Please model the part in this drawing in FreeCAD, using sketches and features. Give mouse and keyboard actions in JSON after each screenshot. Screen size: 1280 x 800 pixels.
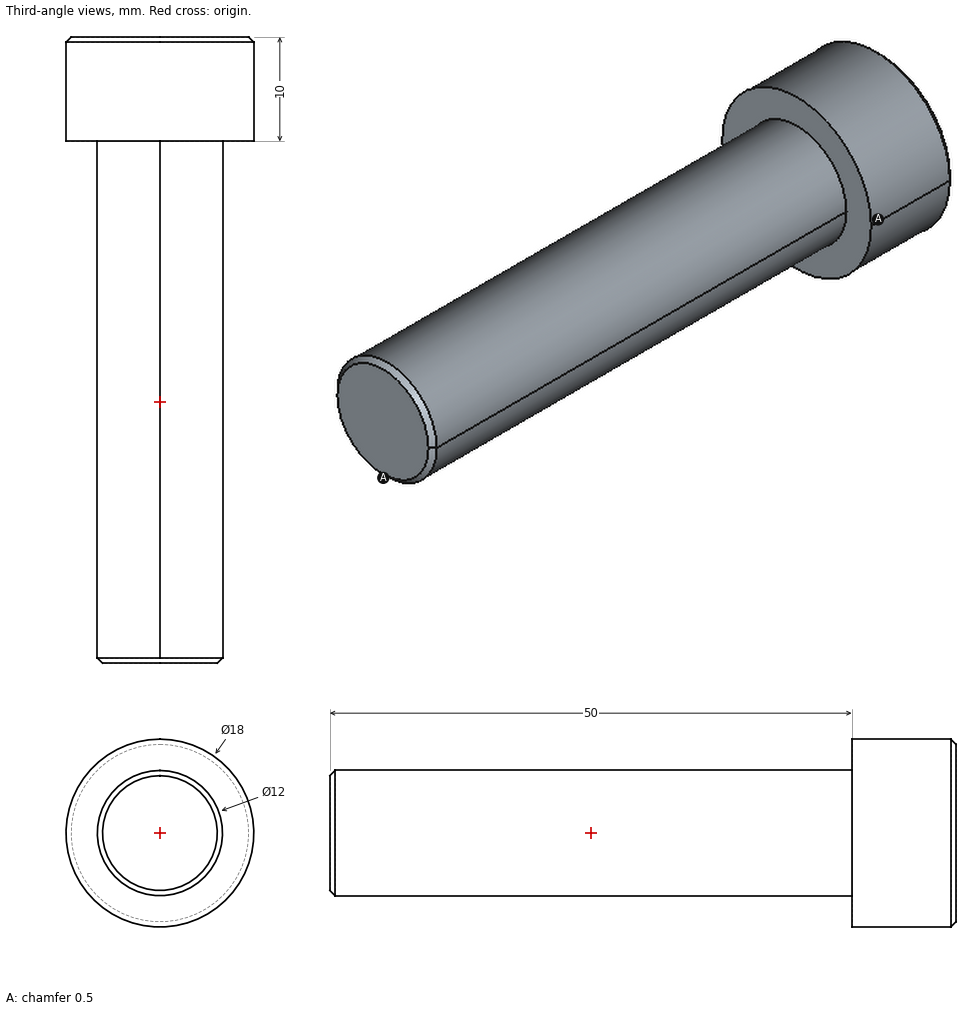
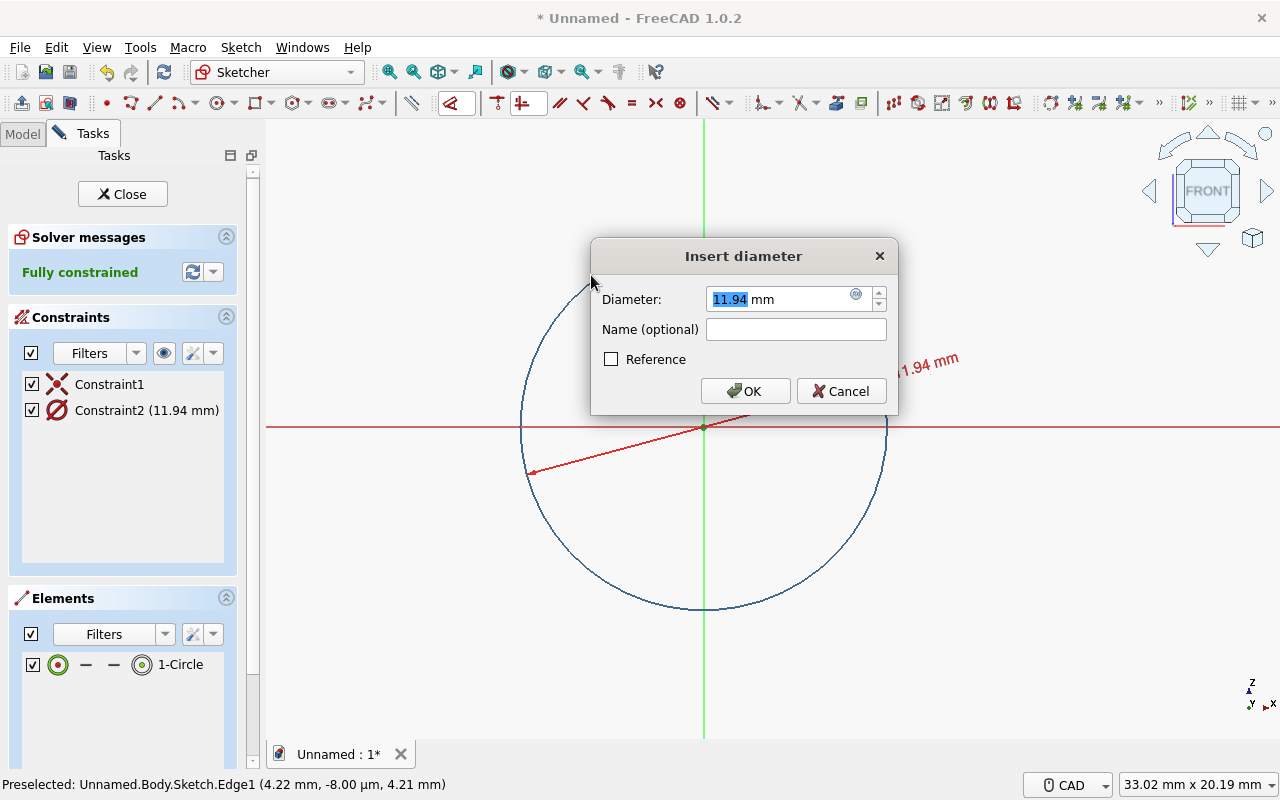
{"action": "type", "text": "12"}
{"action": "key", "text": "Return"}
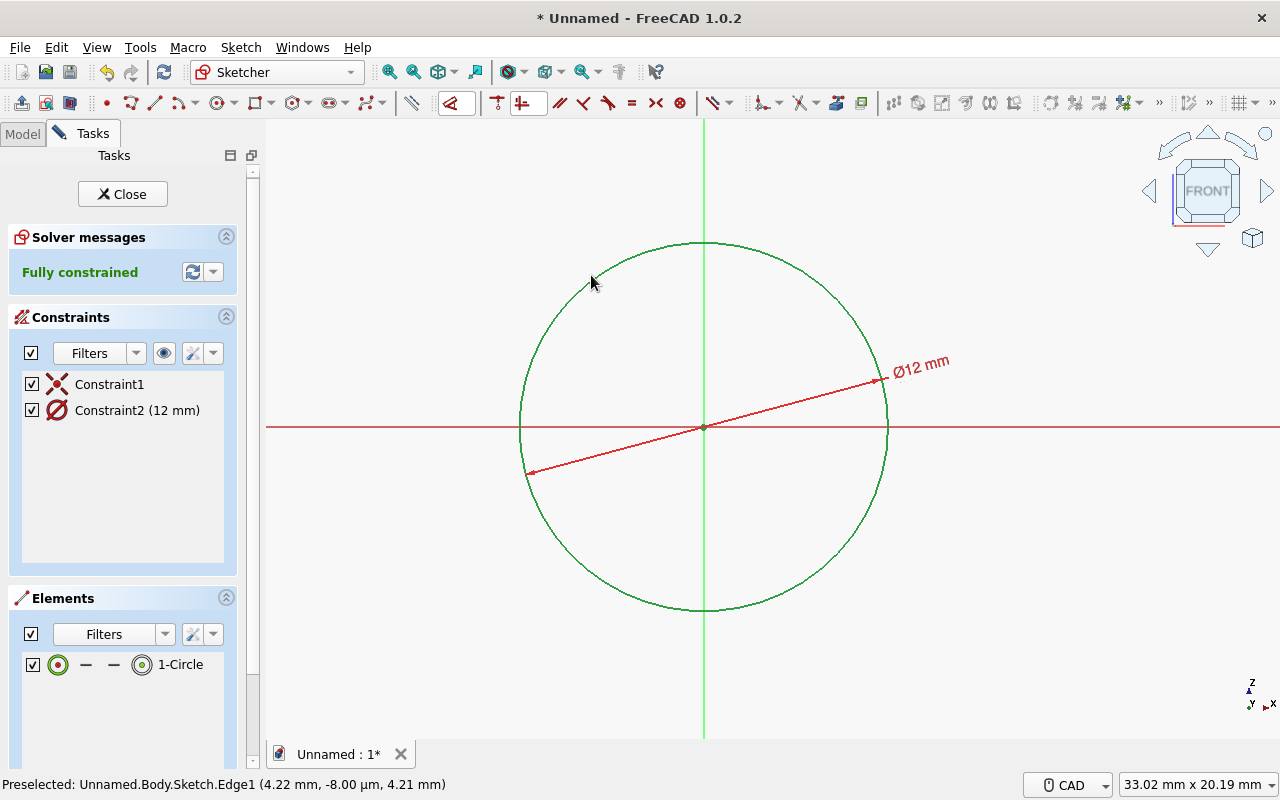
{"action": "left_click", "coordinate": [123, 194]}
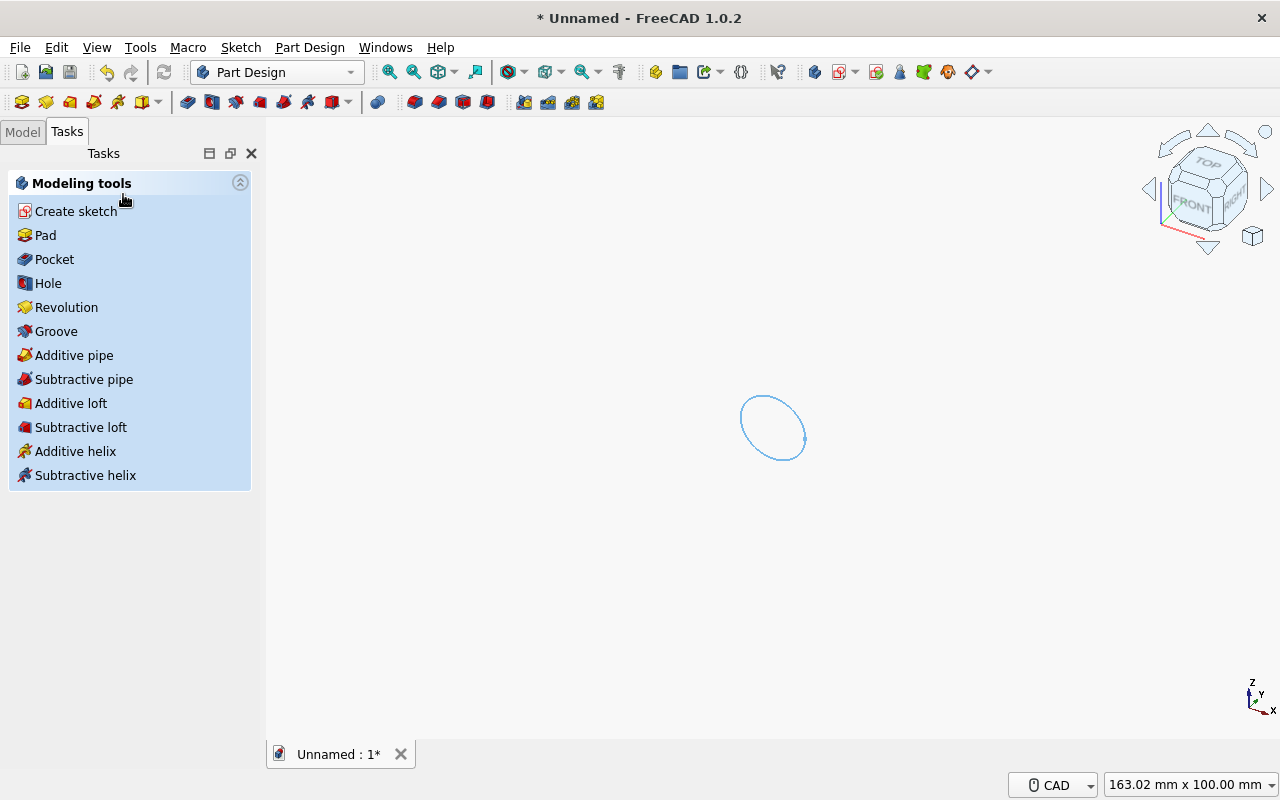
{"action": "left_click", "coordinate": [22, 102]}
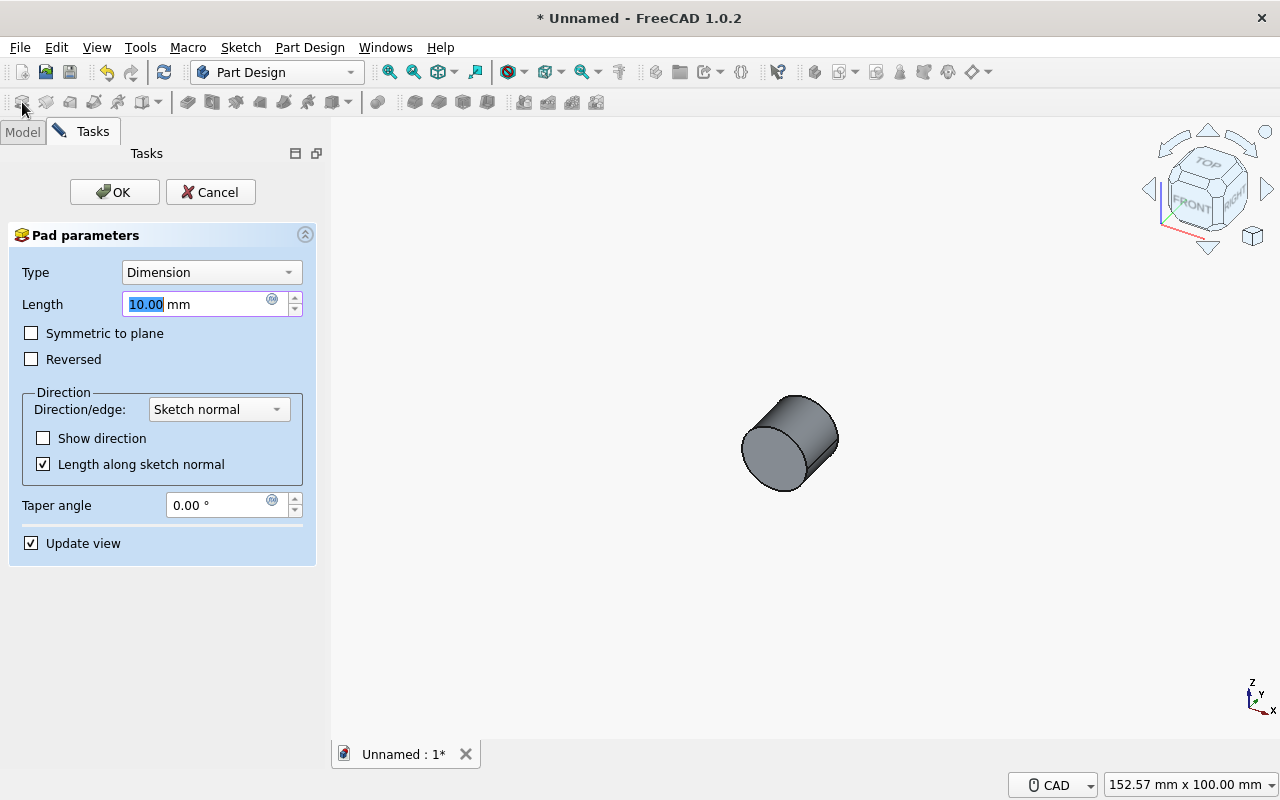
{"action": "type", "text": "50"}
{"action": "key", "text": "Tab"}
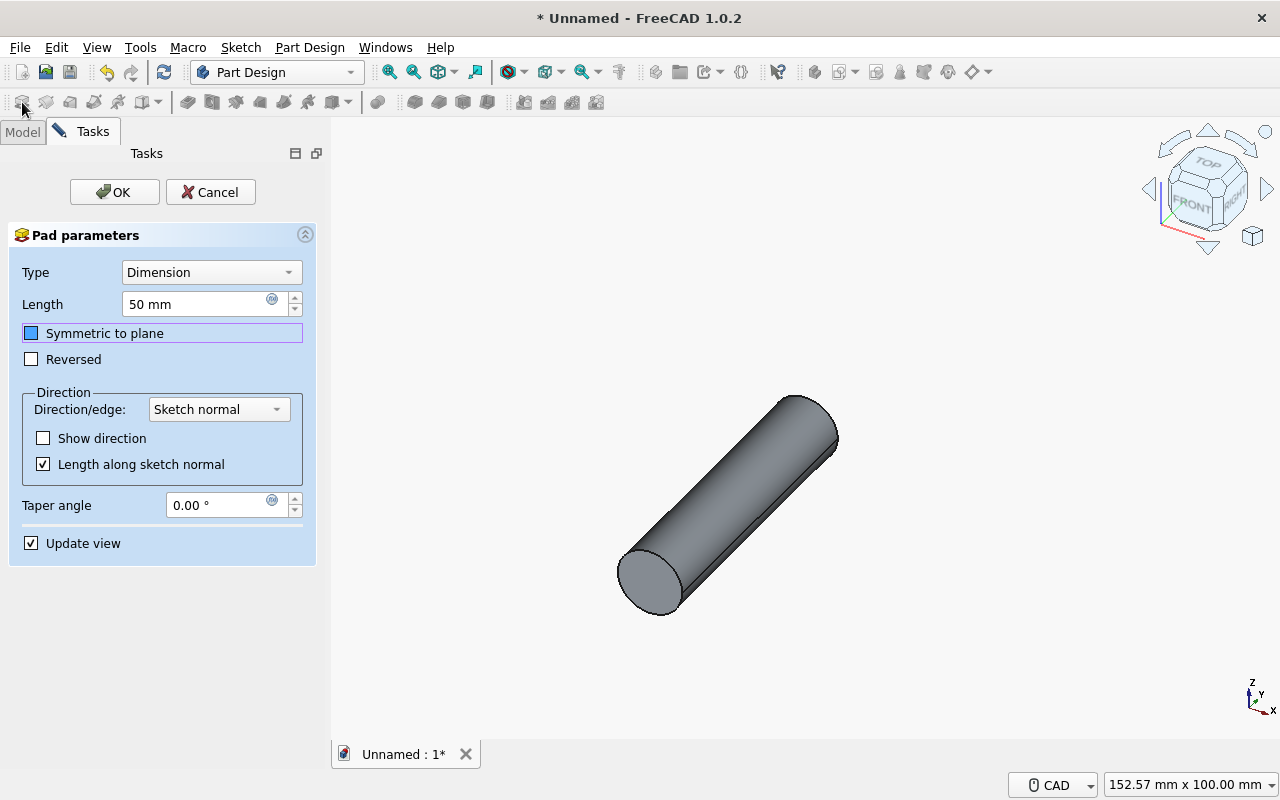
{"action": "left_click", "coordinate": [30, 333]}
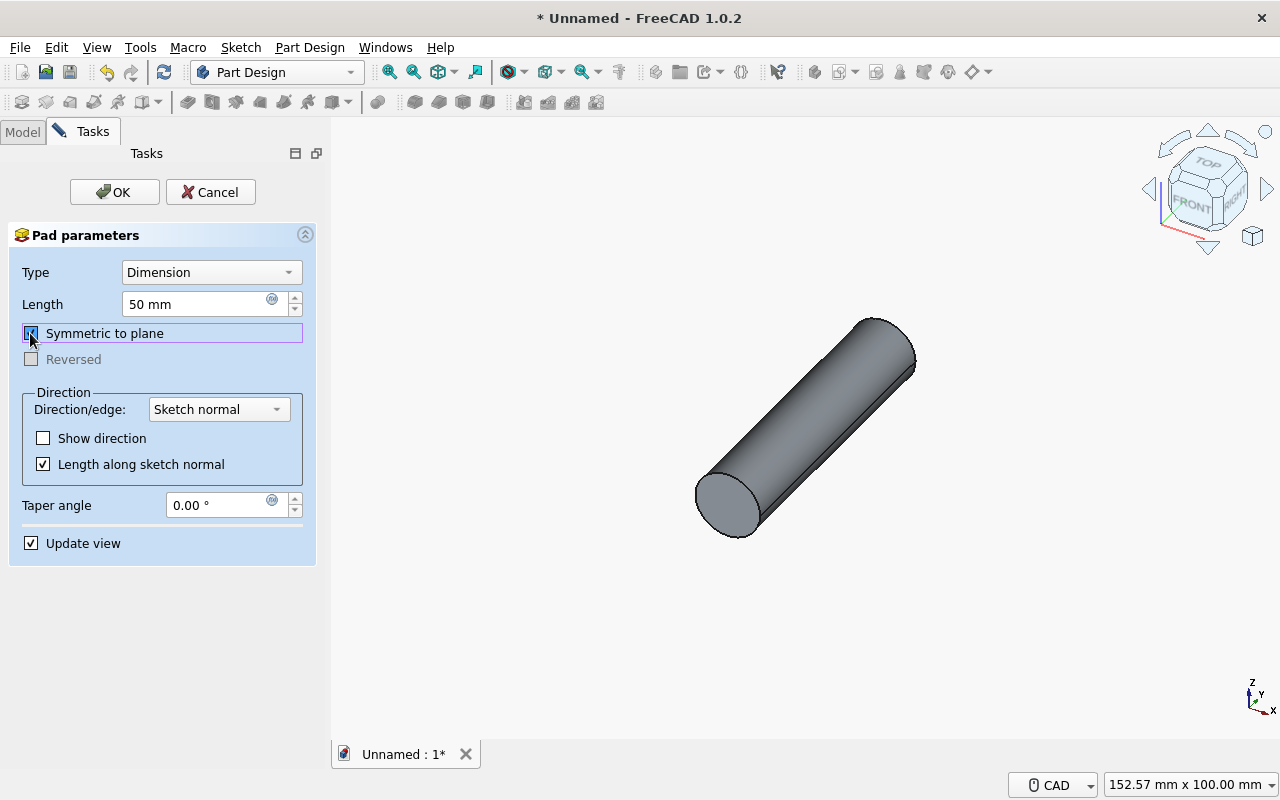
{"action": "left_click", "coordinate": [115, 192]}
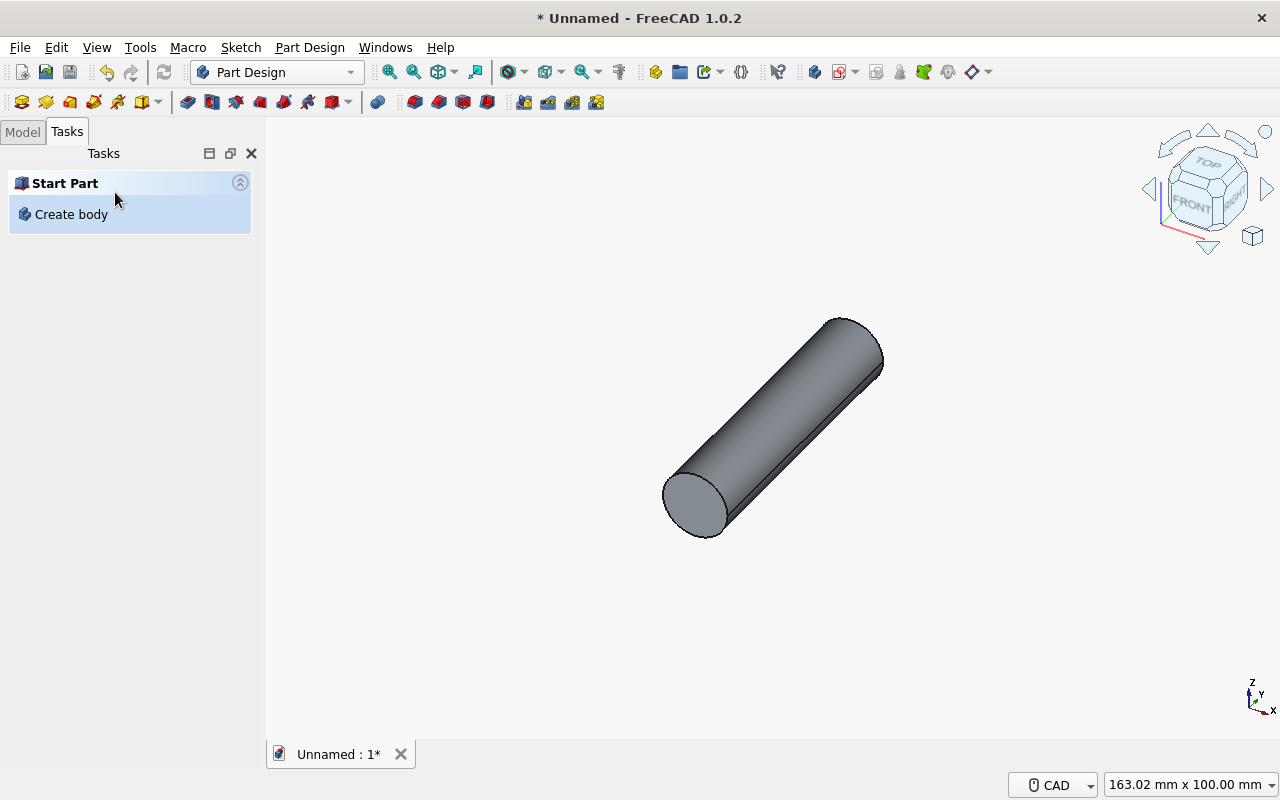
{"action": "left_click", "coordinate": [390, 72]}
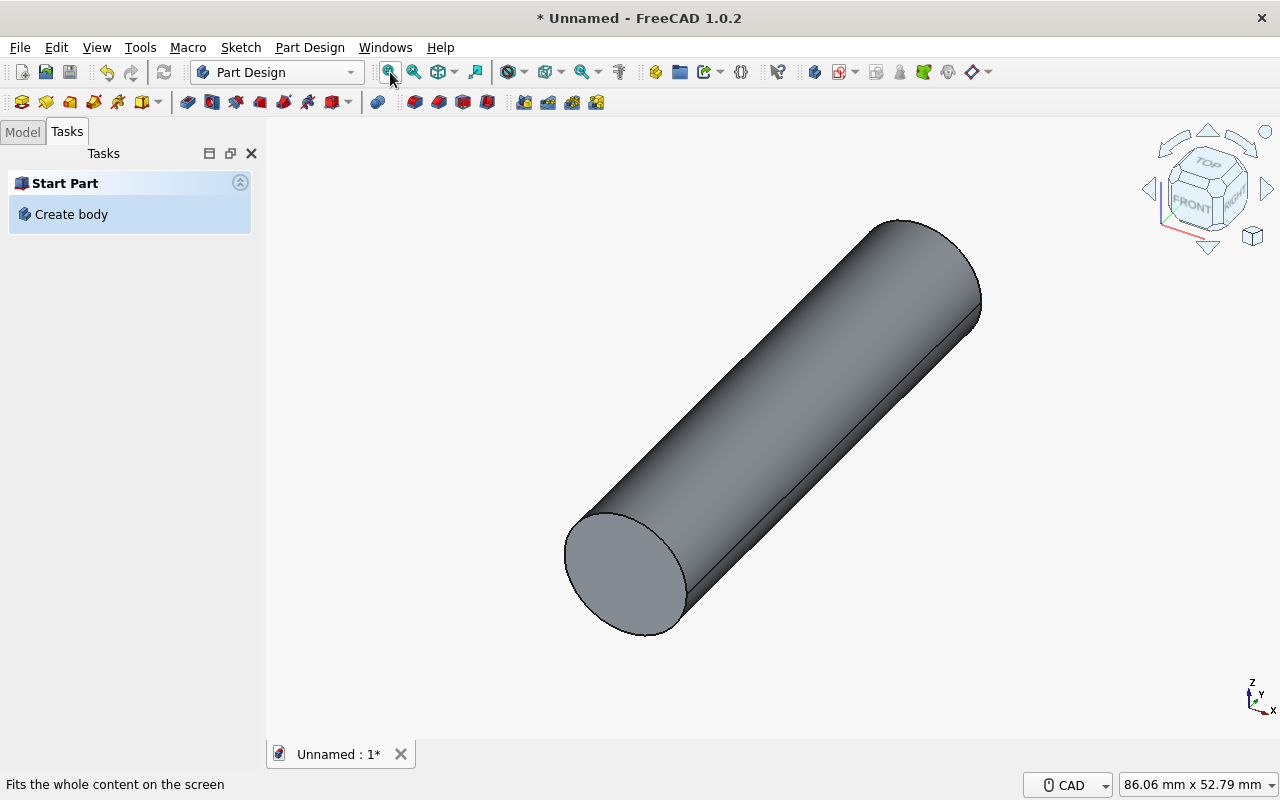
{"action": "key", "text": "4"}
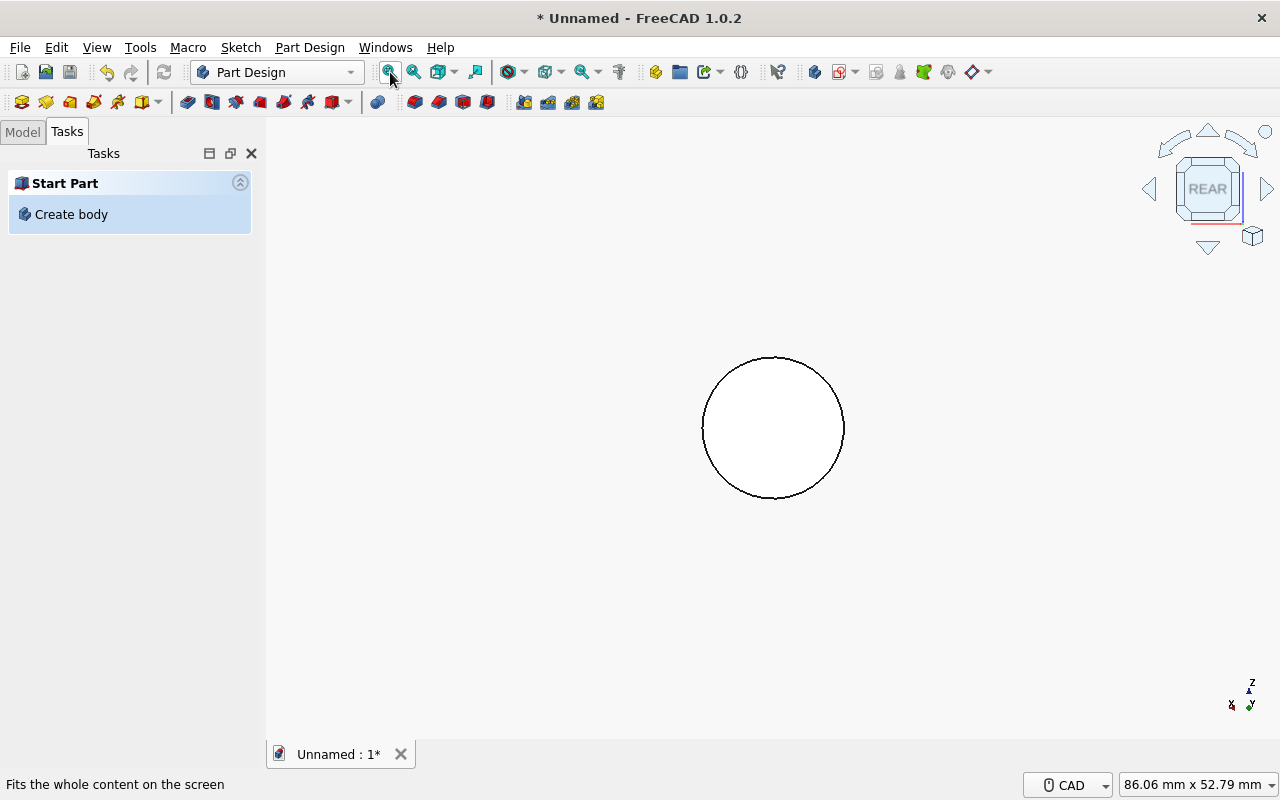
{"action": "left_click", "coordinate": [390, 72]}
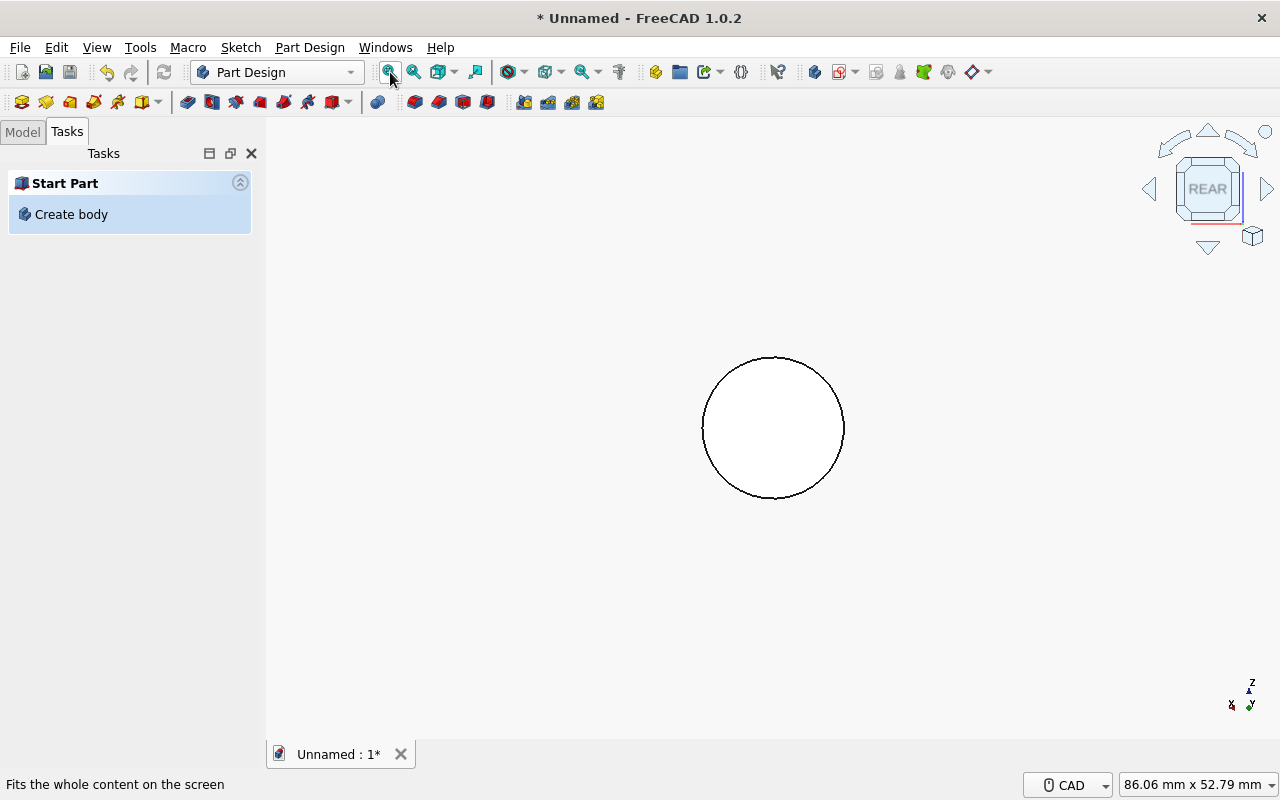
{"action": "left_click", "coordinate": [773, 427]}